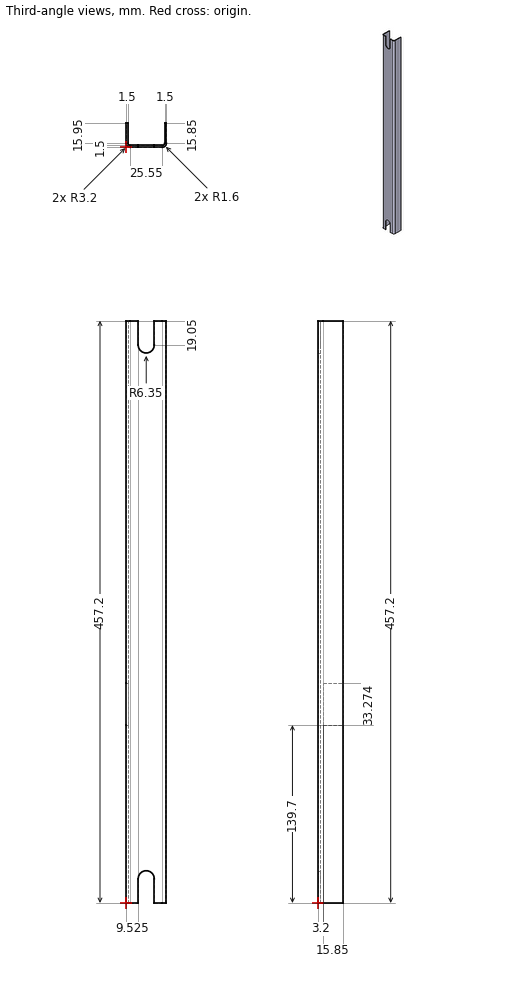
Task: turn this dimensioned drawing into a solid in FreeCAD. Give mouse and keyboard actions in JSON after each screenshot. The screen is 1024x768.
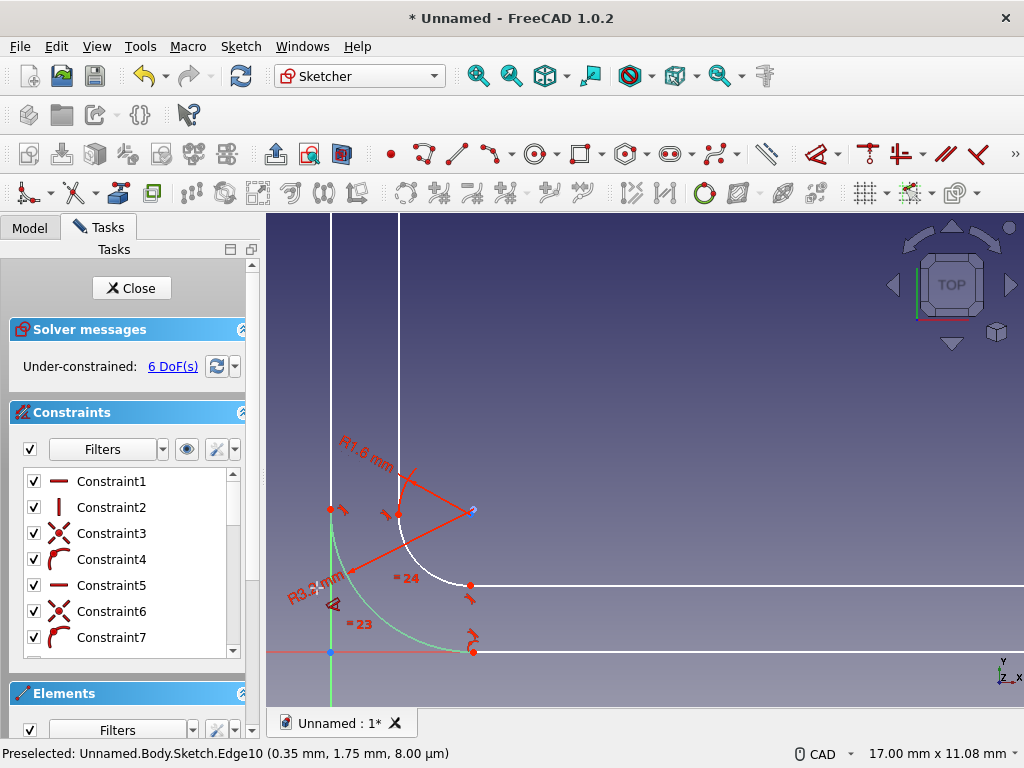
{"action": "scroll", "coordinate": [377, 560], "scroll_direction": "down", "scroll_amount": 6}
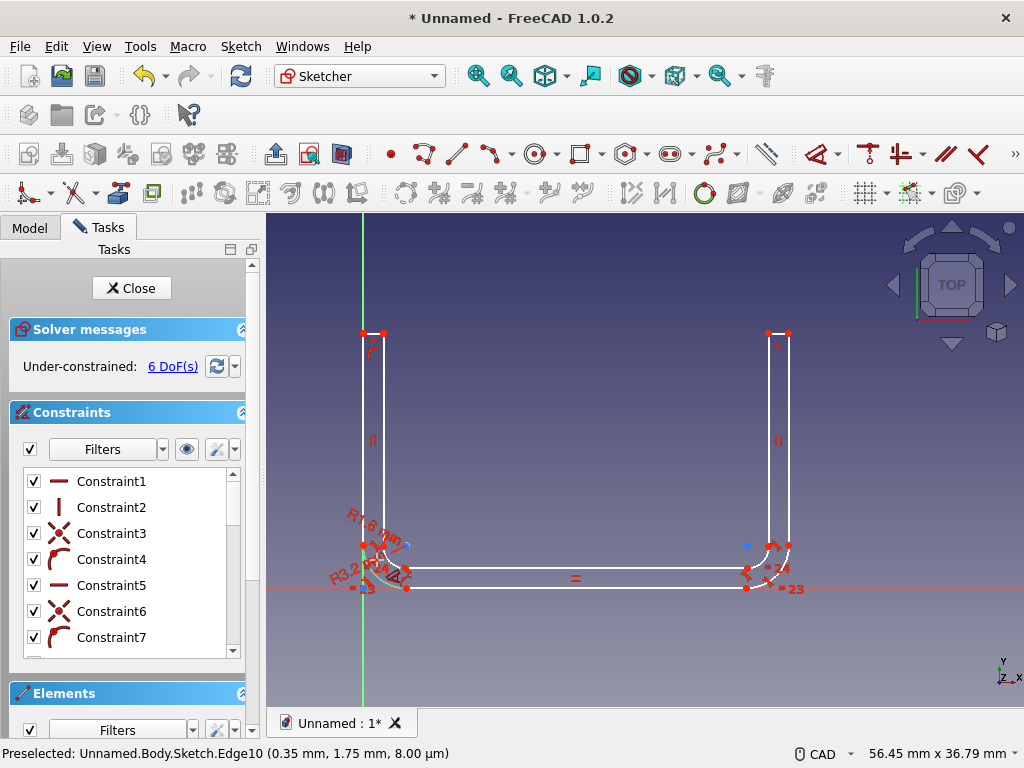
{"action": "scroll", "coordinate": [378, 334], "scroll_direction": "up", "scroll_amount": 5}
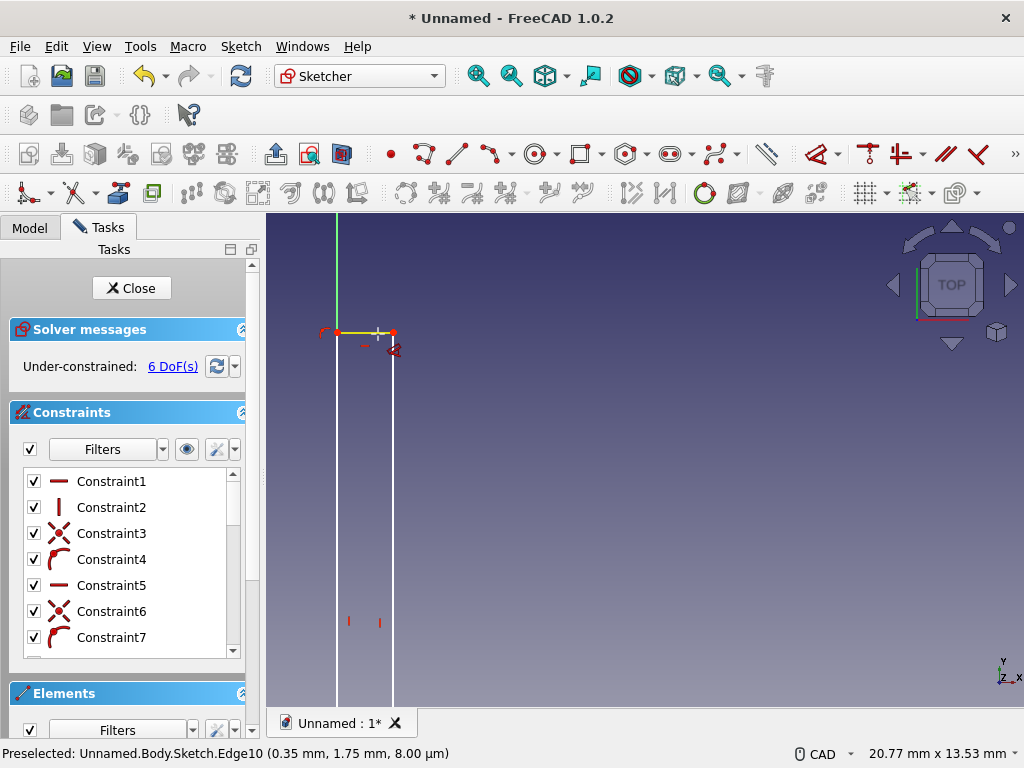
{"action": "left_click", "coordinate": [376, 333]}
{"action": "left_click", "coordinate": [365, 299]}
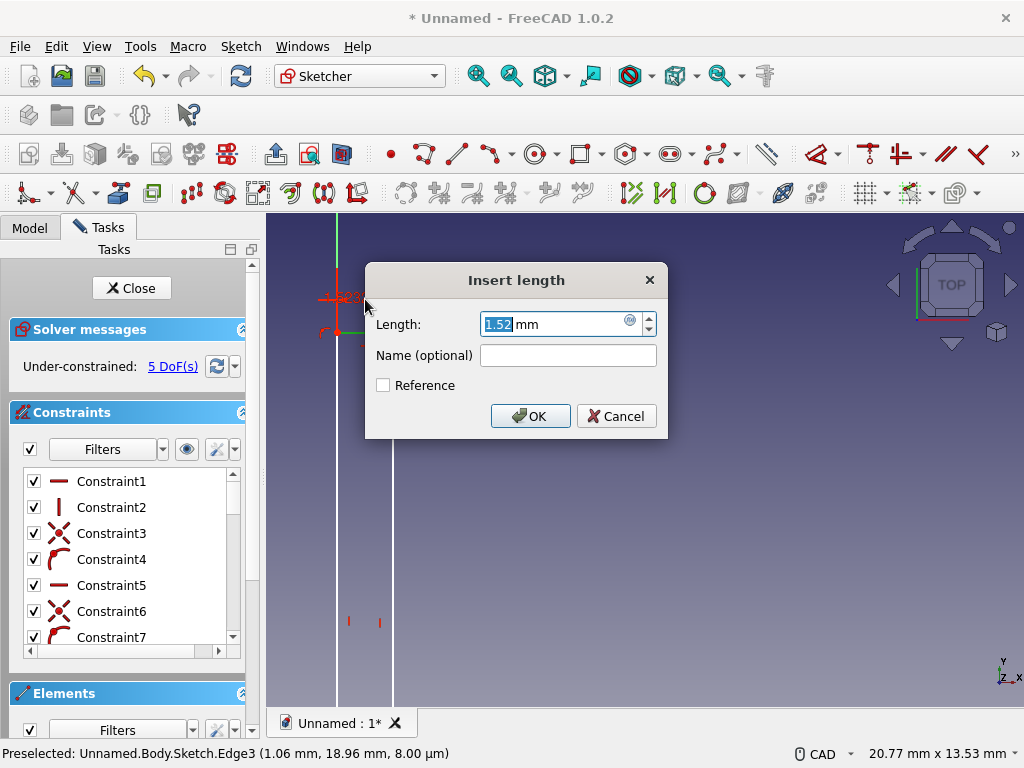
{"action": "type", "text": "1.5"}
{"action": "key", "text": "Return"}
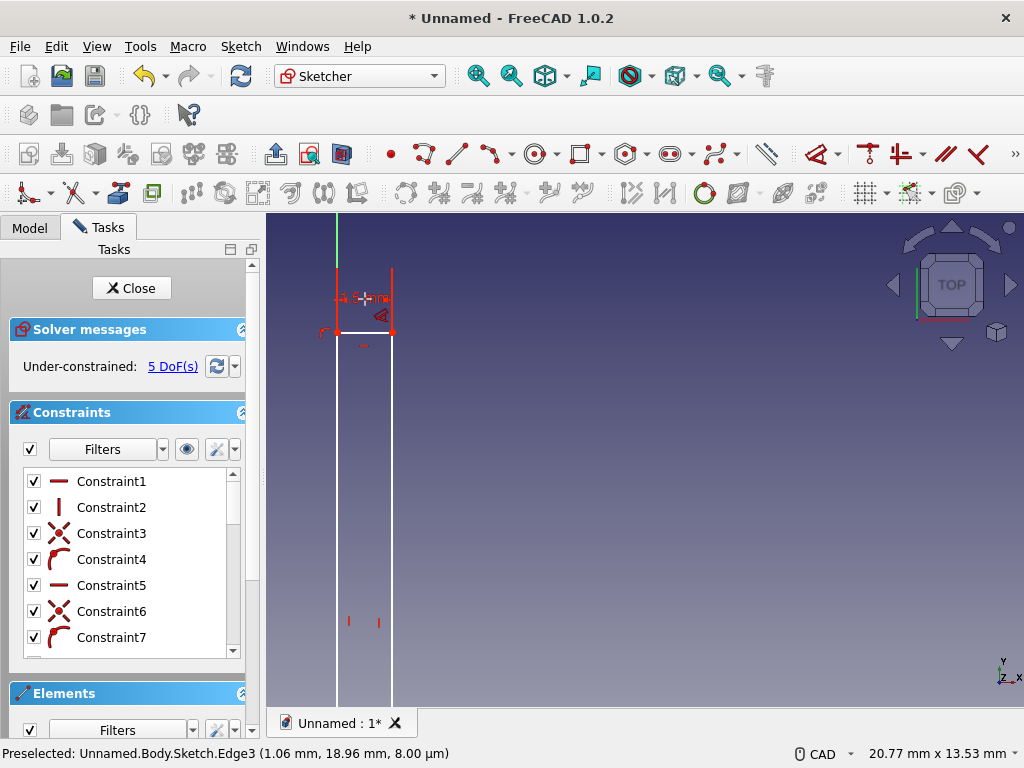
{"action": "scroll", "coordinate": [378, 334], "scroll_direction": "down", "scroll_amount": 5}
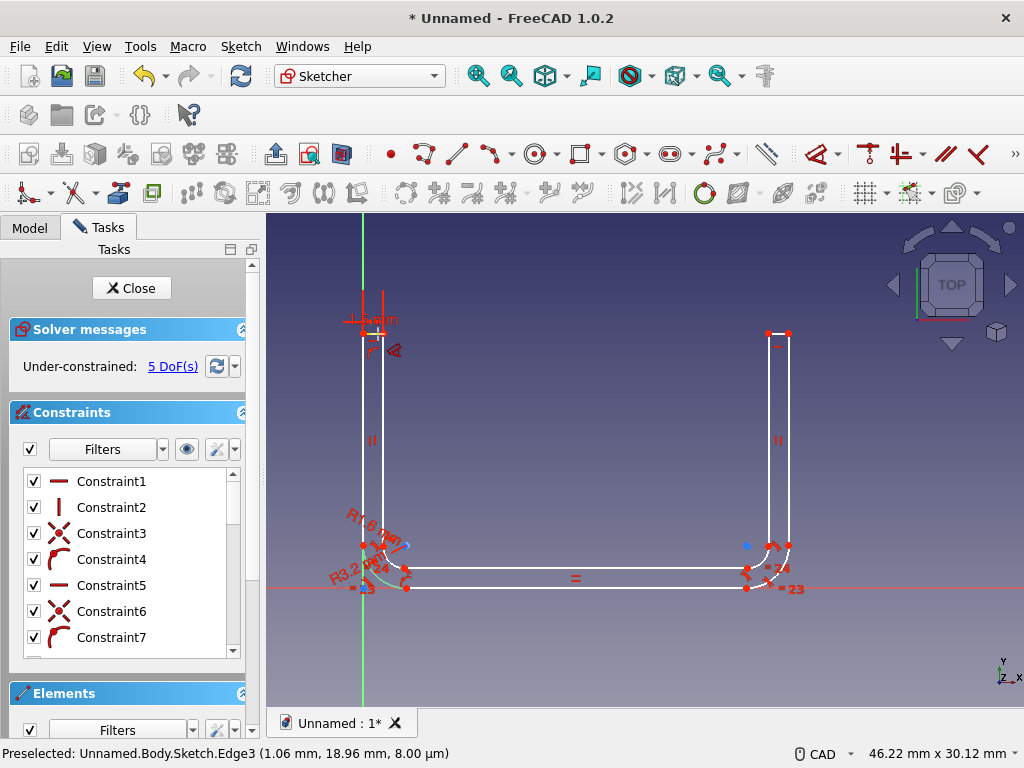
{"action": "scroll", "coordinate": [783, 334], "scroll_direction": "up", "scroll_amount": 5}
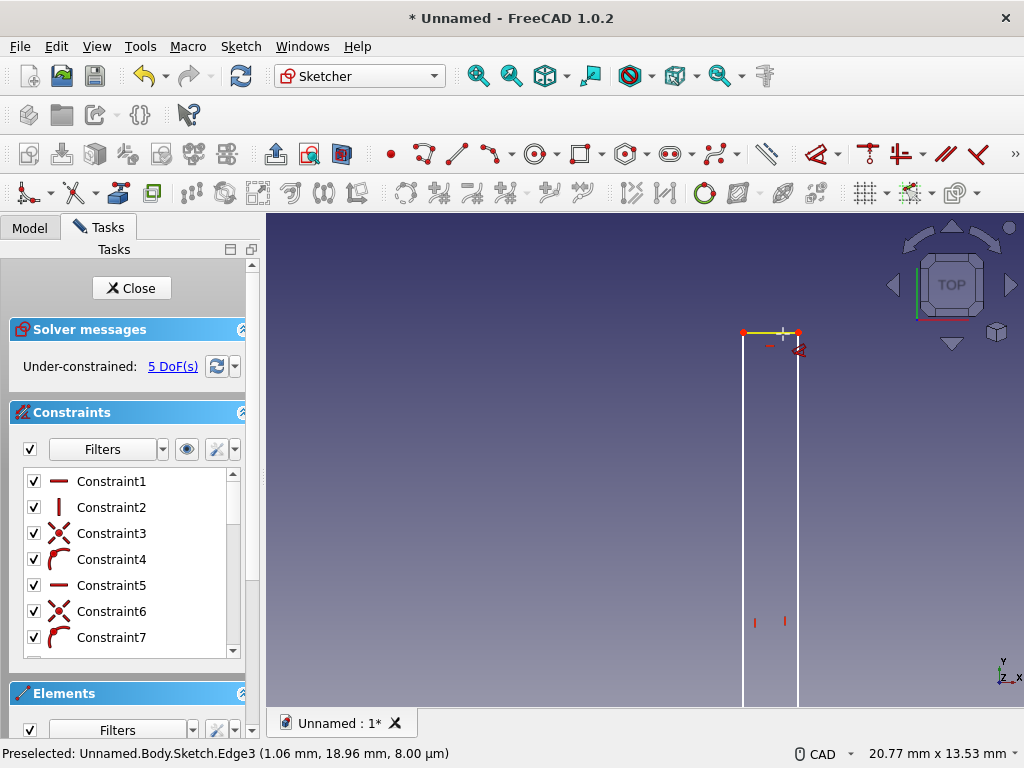
{"action": "left_click", "coordinate": [782, 333]}
{"action": "left_click", "coordinate": [771, 299]}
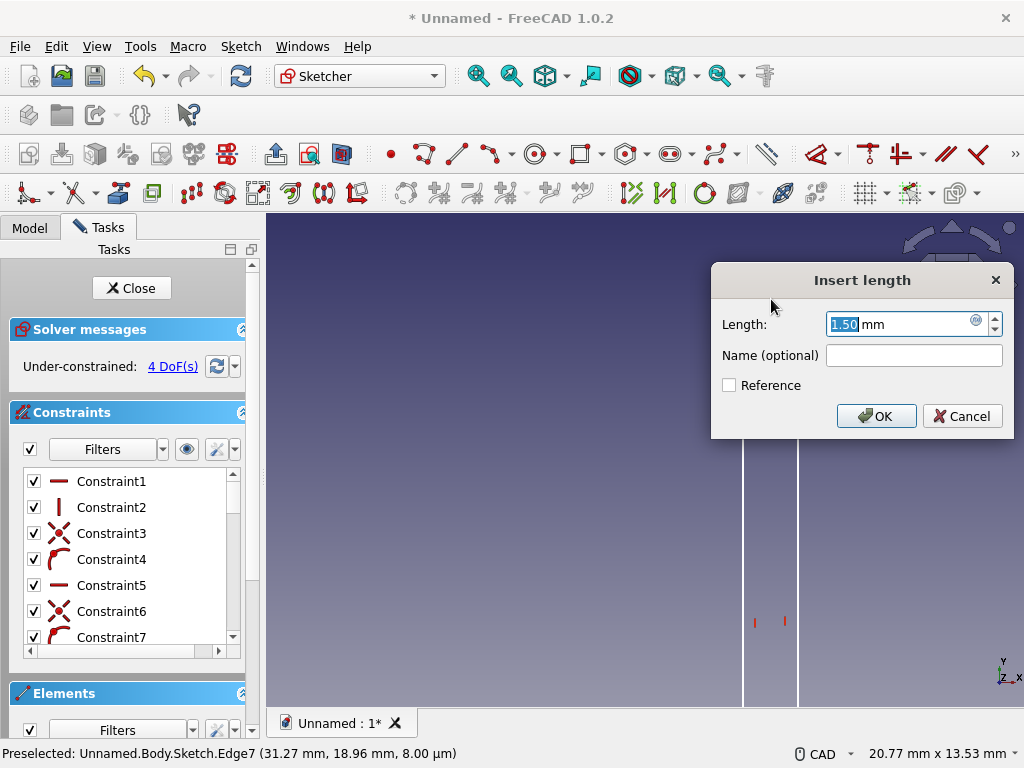
{"action": "type", "text": "1.5"}
{"action": "key", "text": "Return"}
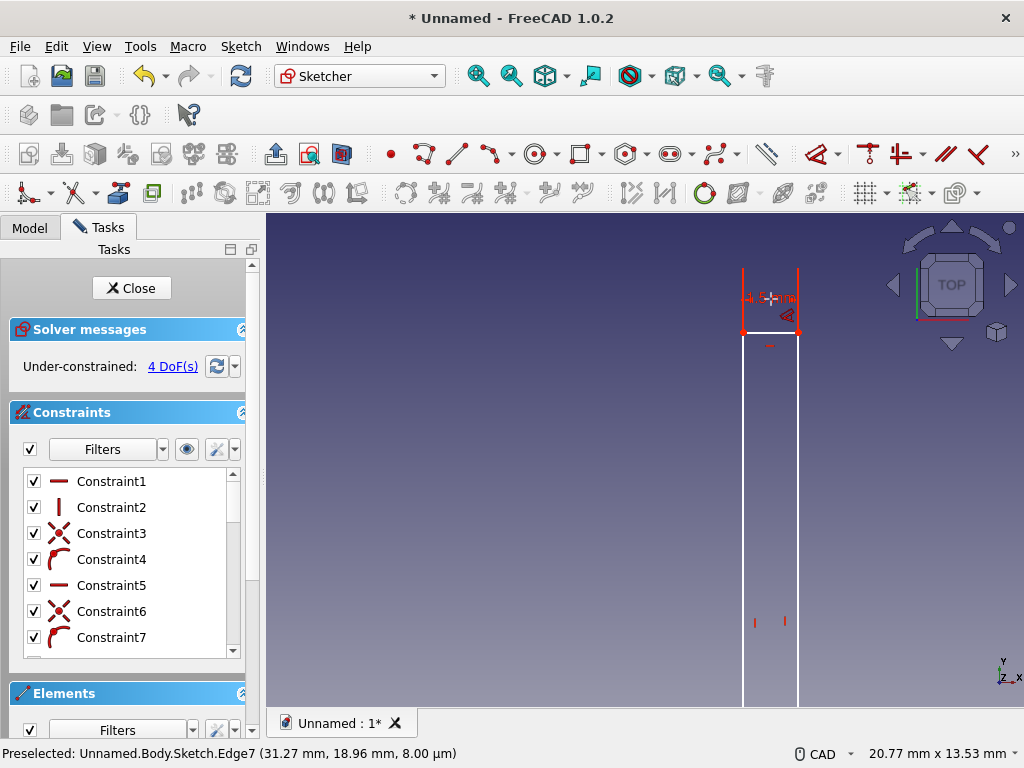
{"action": "scroll", "coordinate": [784, 334], "scroll_direction": "down", "scroll_amount": 5}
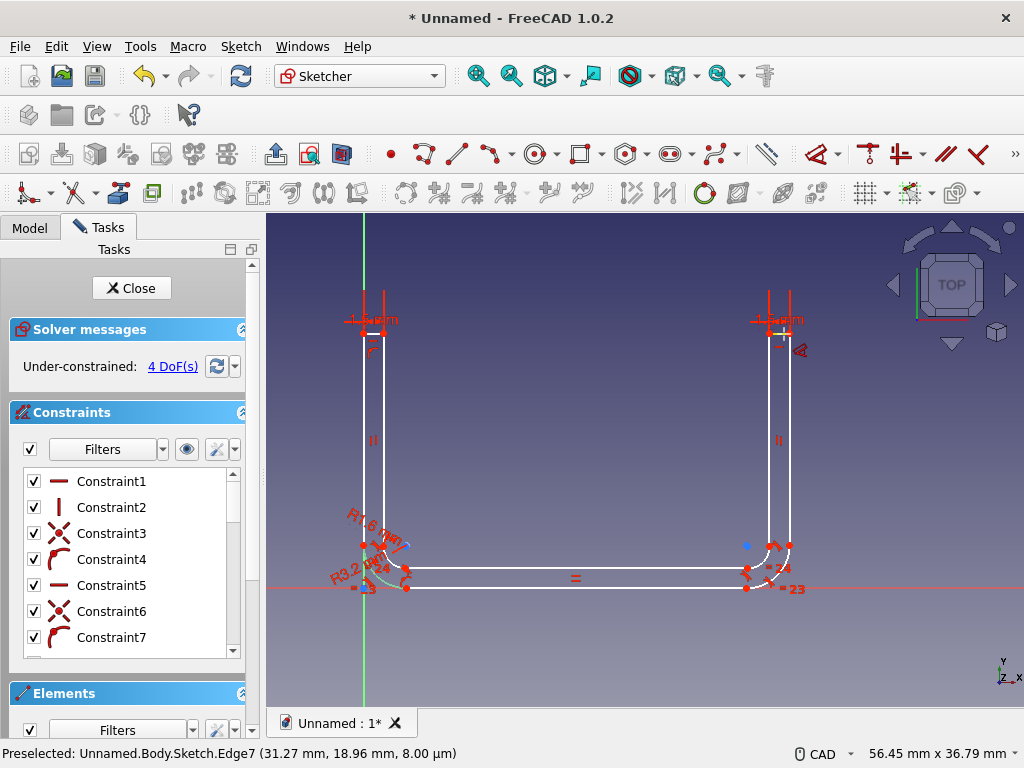
{"action": "scroll", "coordinate": [748, 568], "scroll_direction": "up", "scroll_amount": 4}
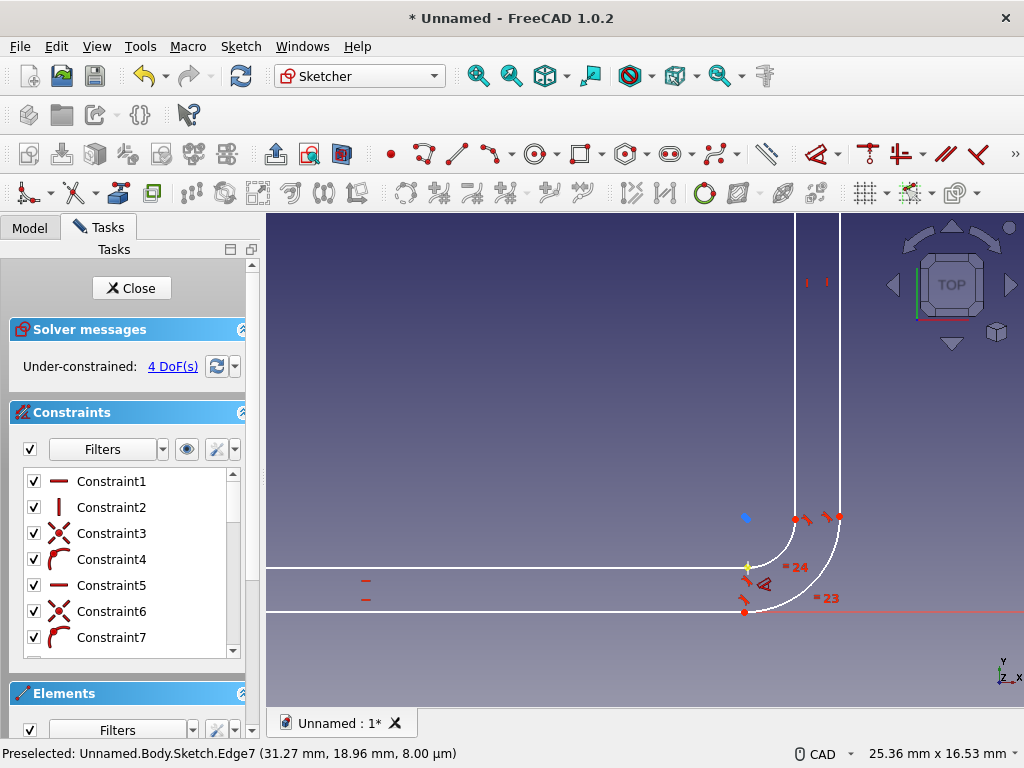
{"action": "left_click", "coordinate": [747, 568]}
{"action": "left_click", "coordinate": [781, 590]}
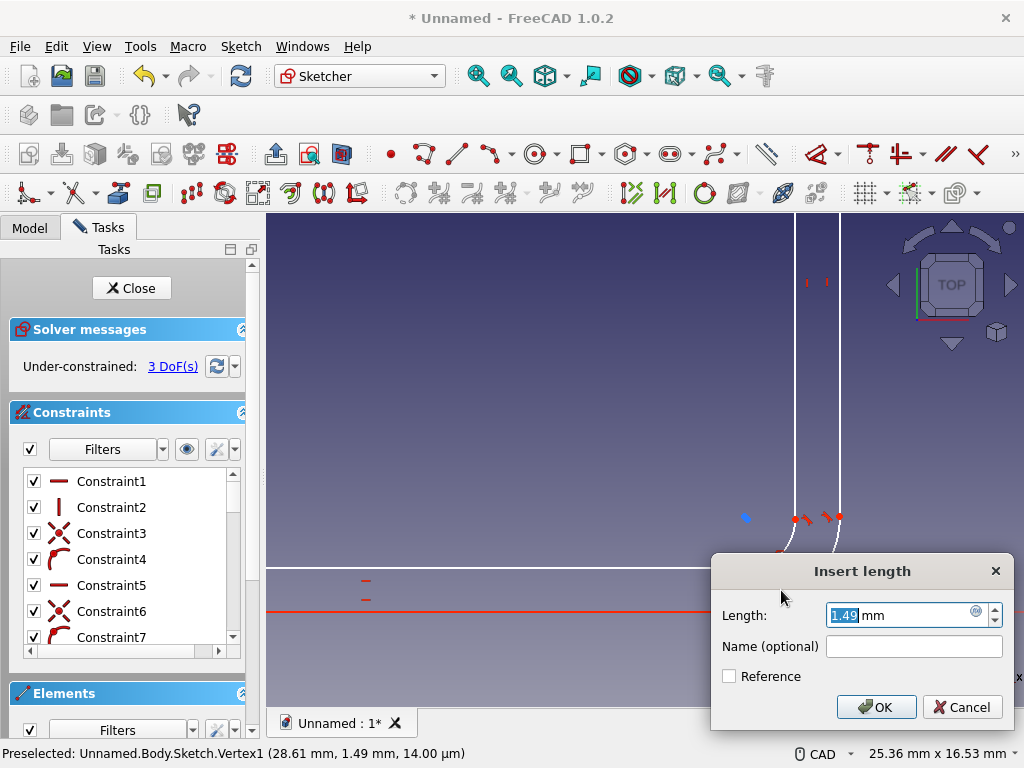
{"action": "type", "text": "1.5"}
{"action": "key", "text": "Return"}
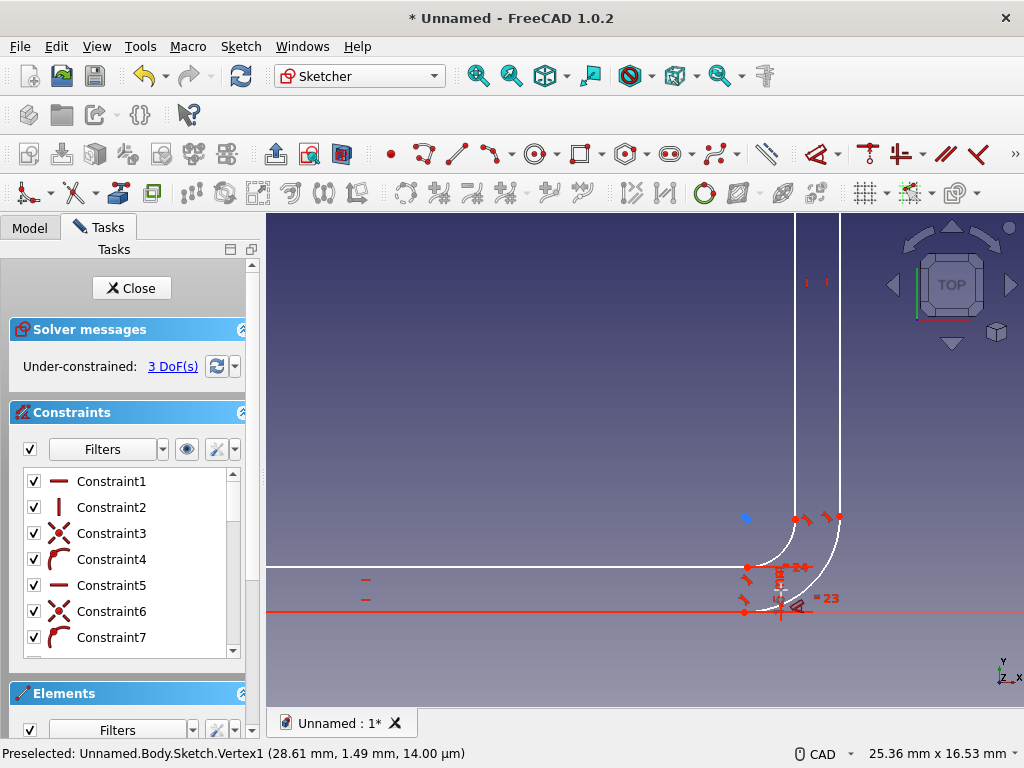
{"action": "left_click", "coordinate": [518, 567]}
{"action": "left_click", "coordinate": [521, 533]}